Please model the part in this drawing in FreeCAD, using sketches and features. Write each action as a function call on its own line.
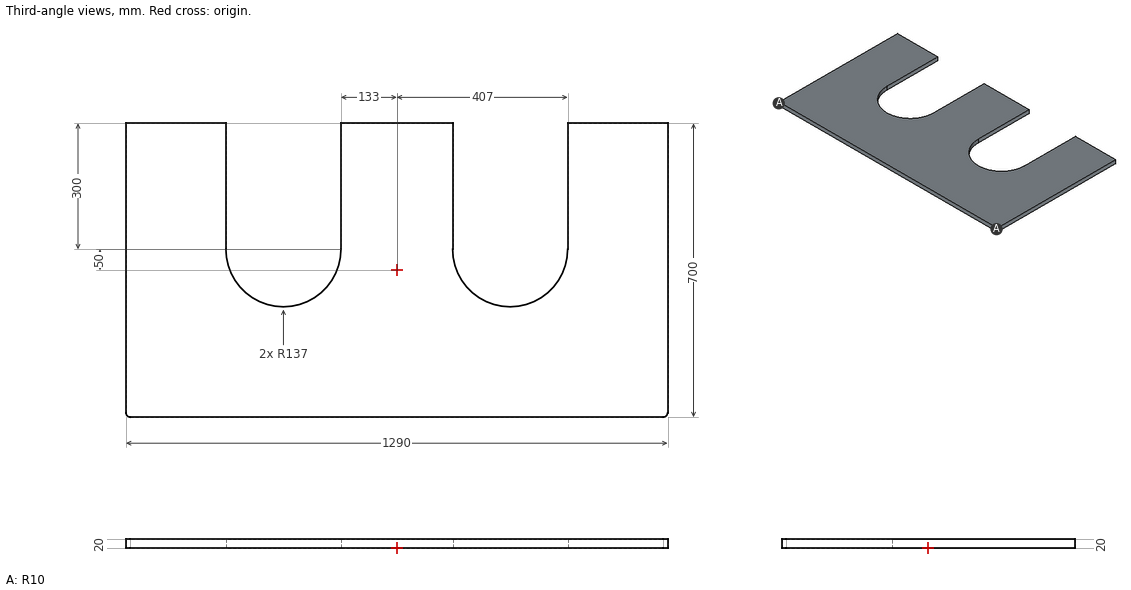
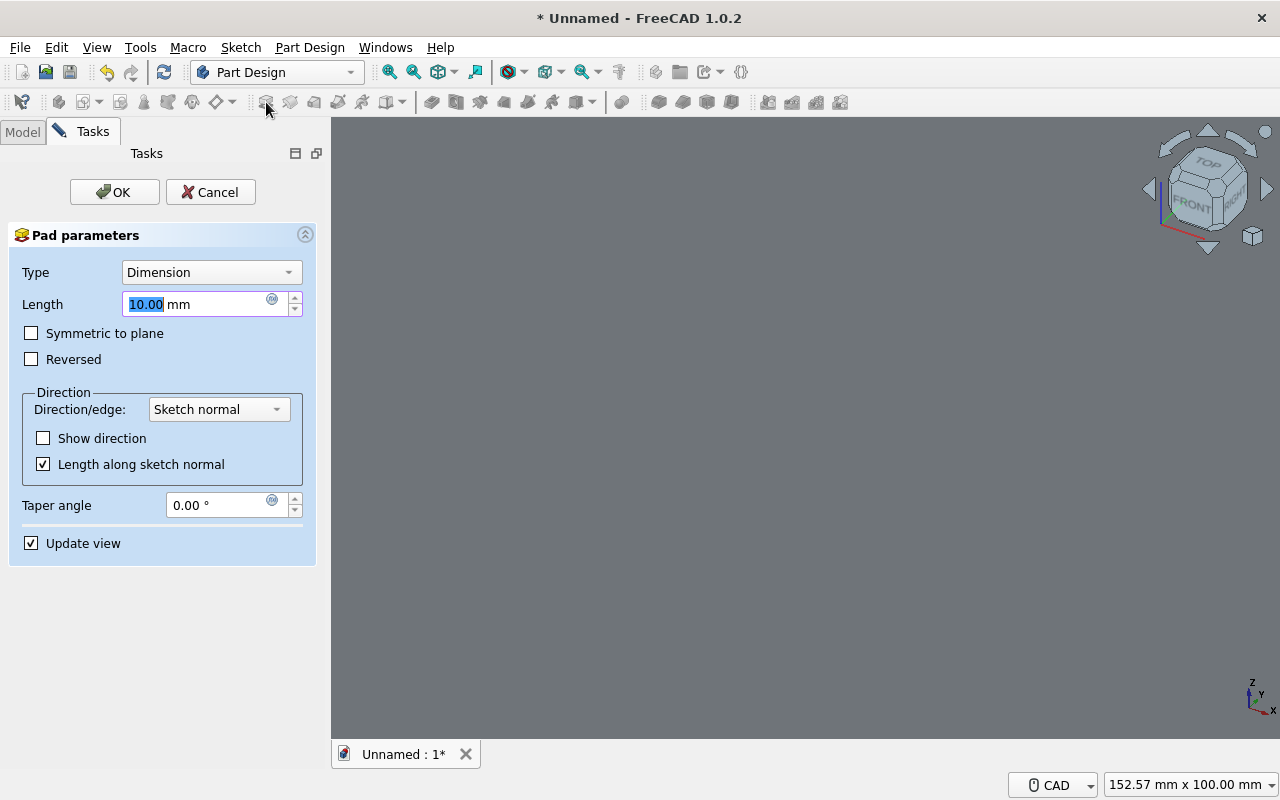
text(20)
key(Tab)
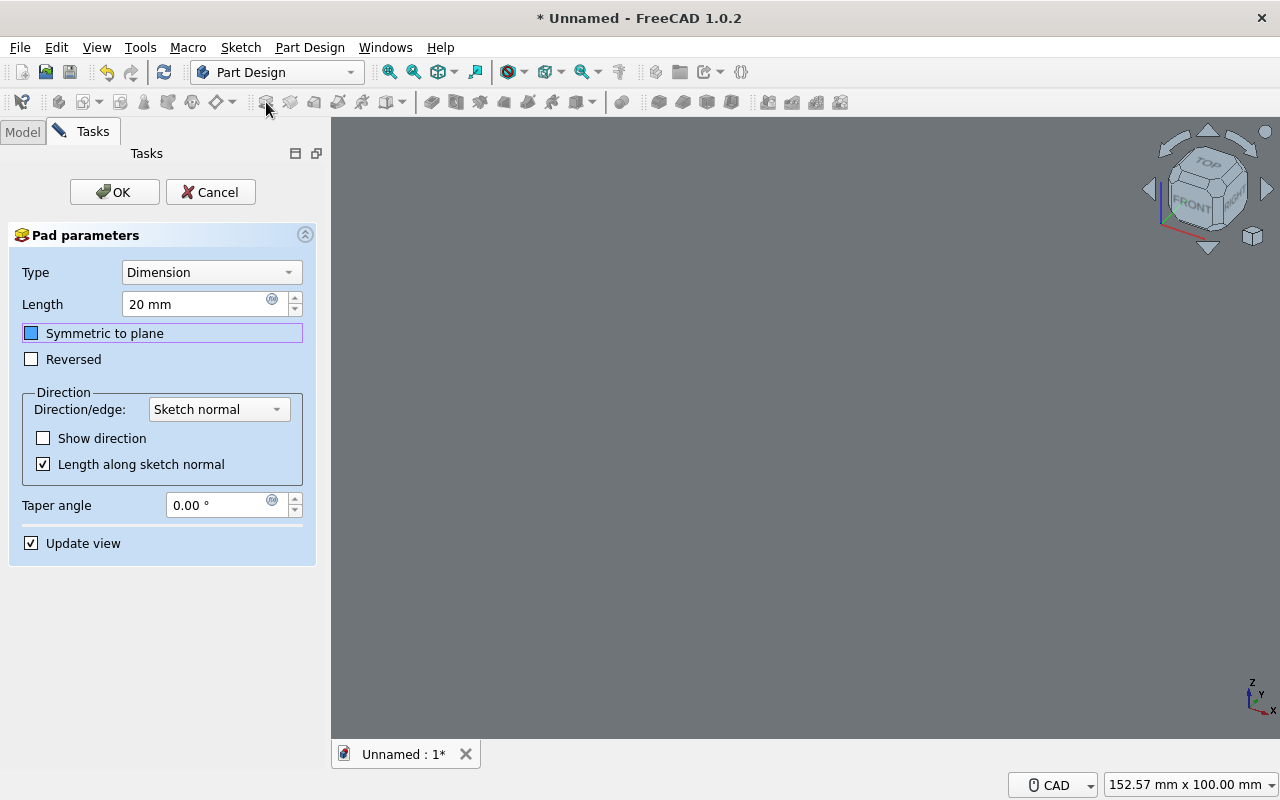
click(115, 192)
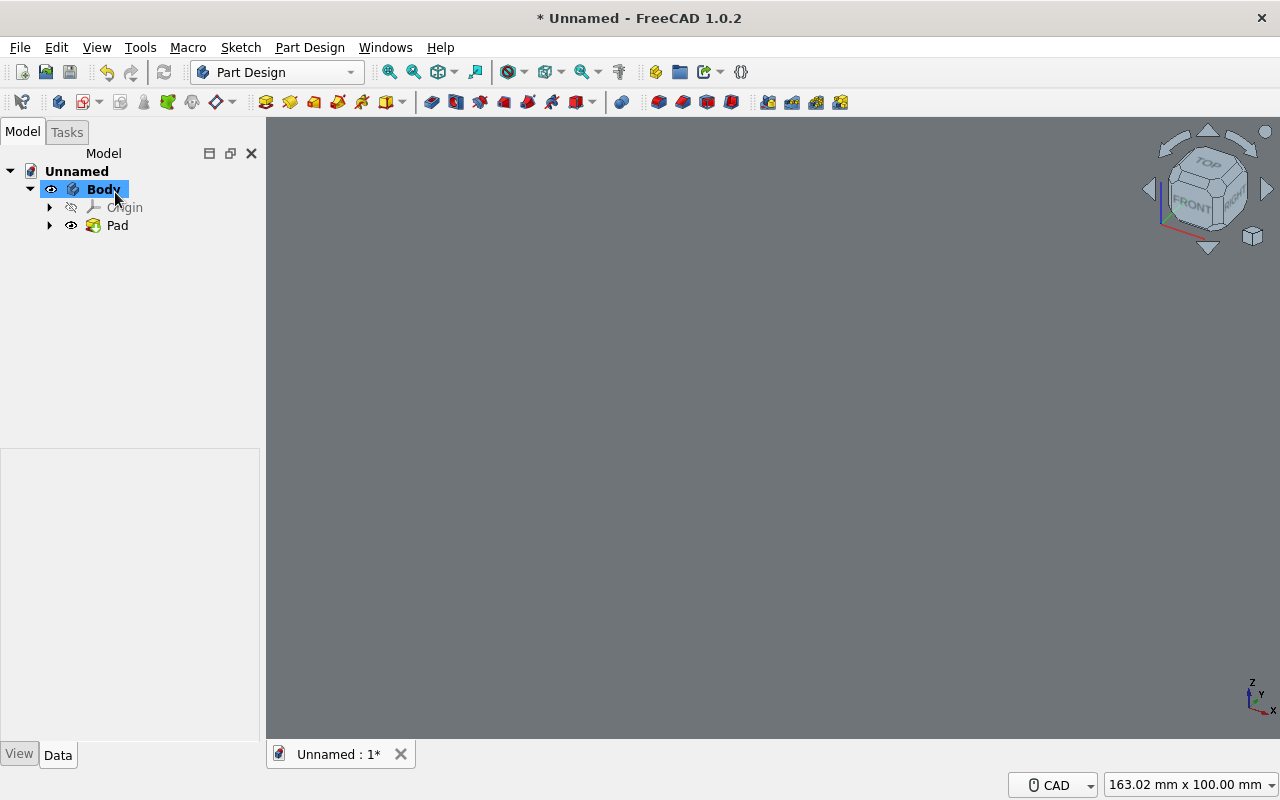
key(v)
key(f)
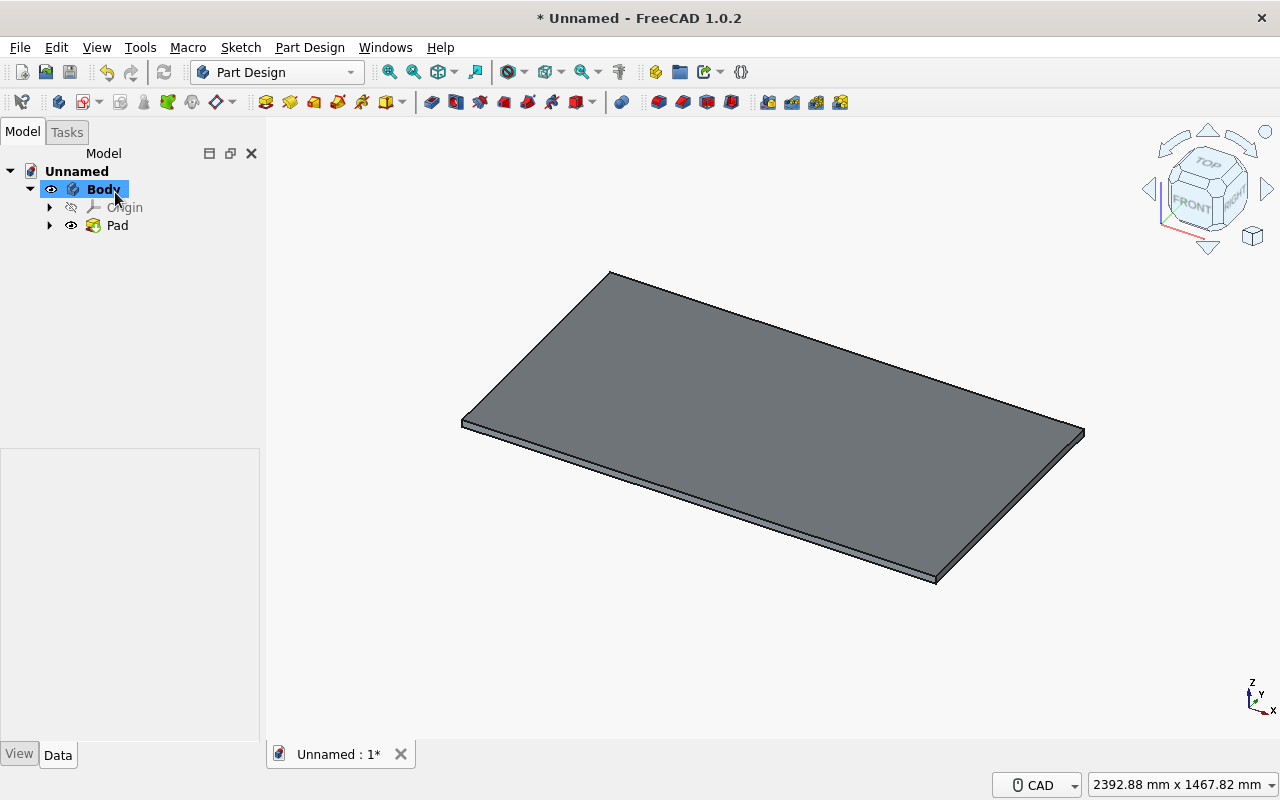
click(841, 446)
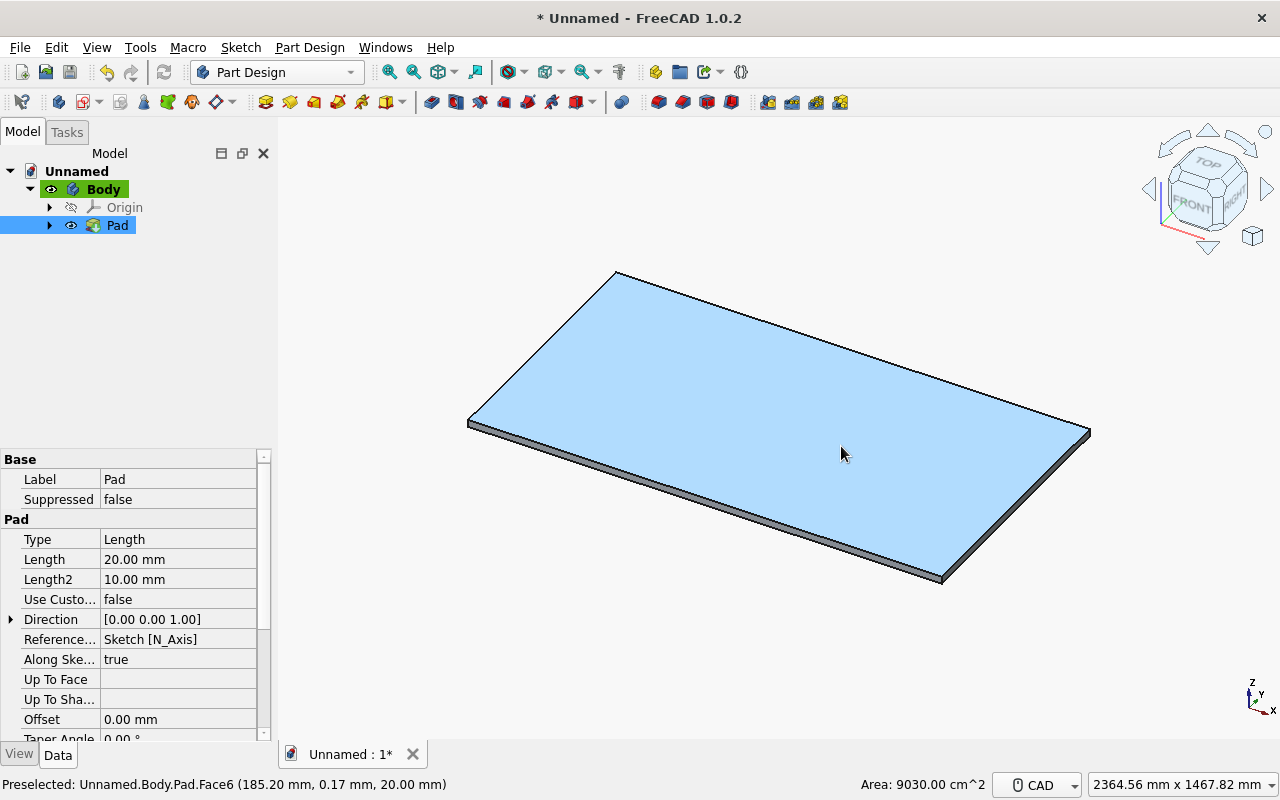
click(84, 102)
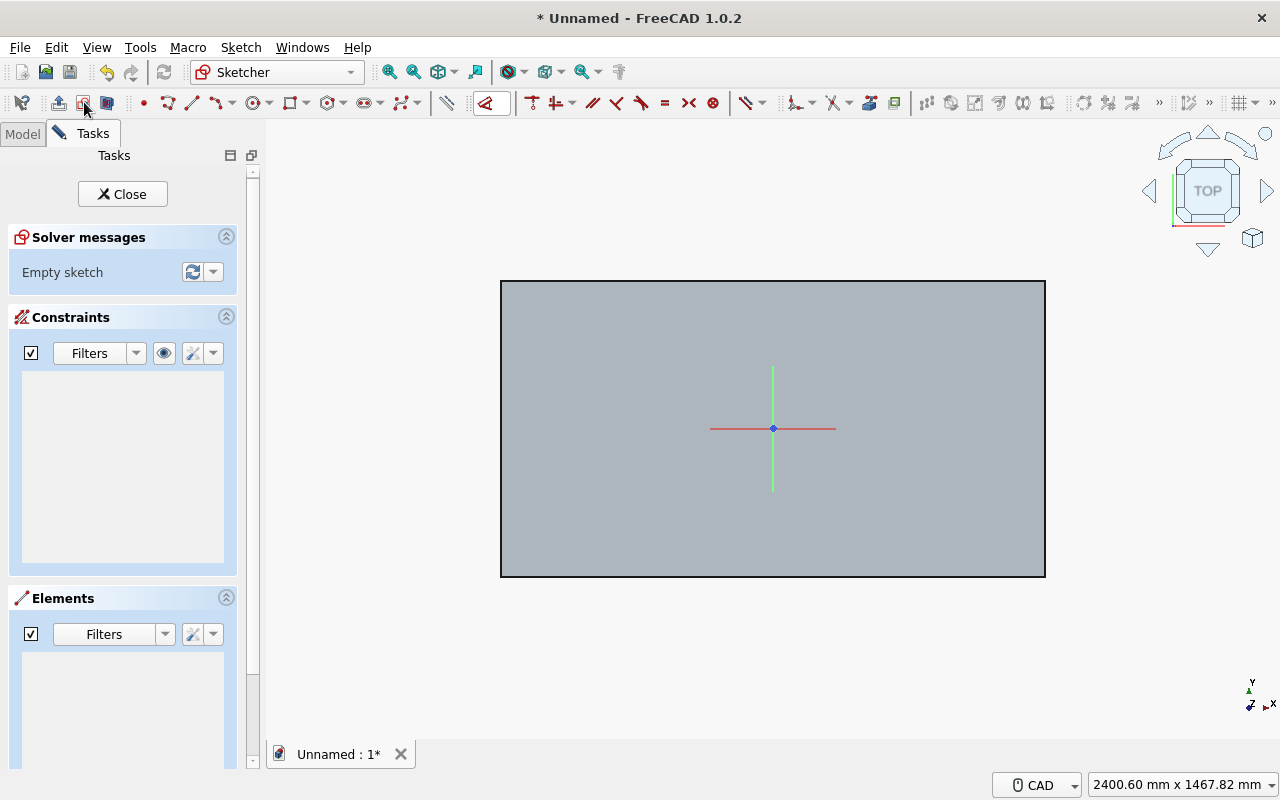
scroll(856, 306, up, 3)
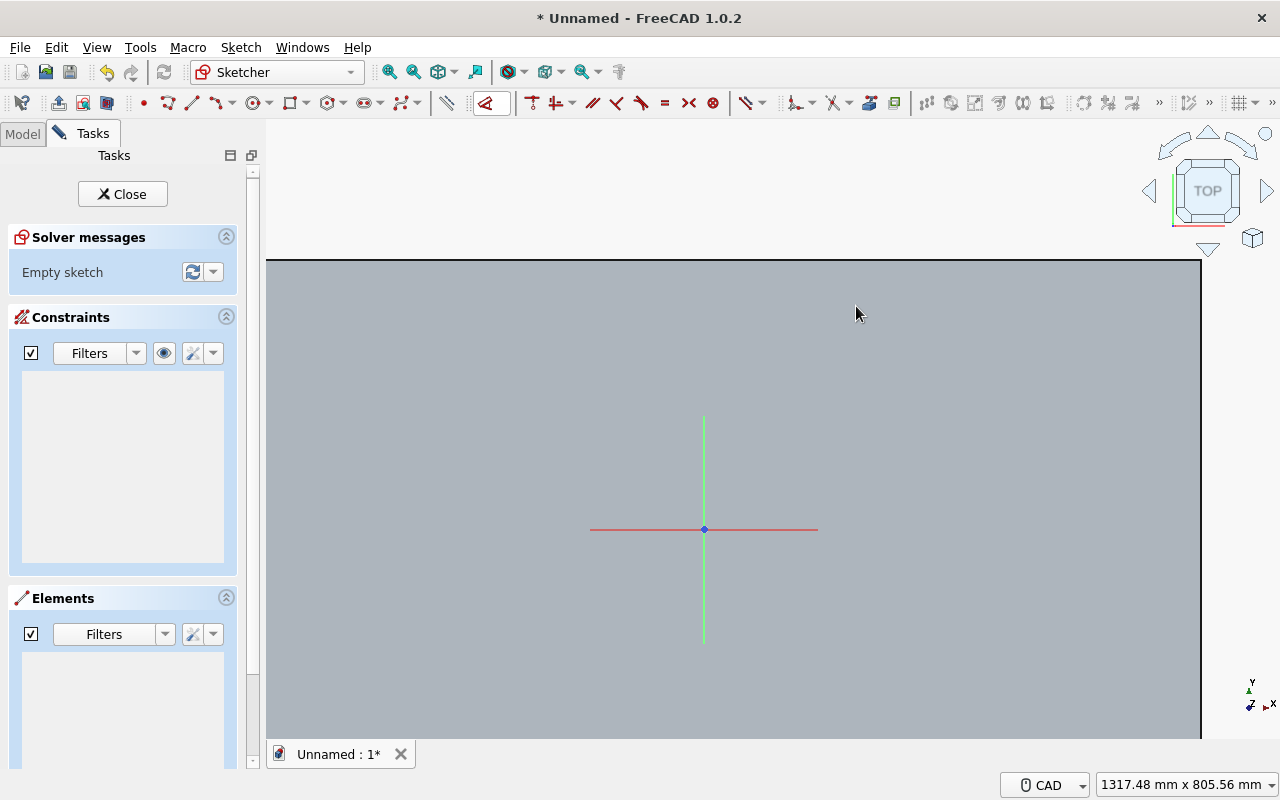
key(g)
key(m)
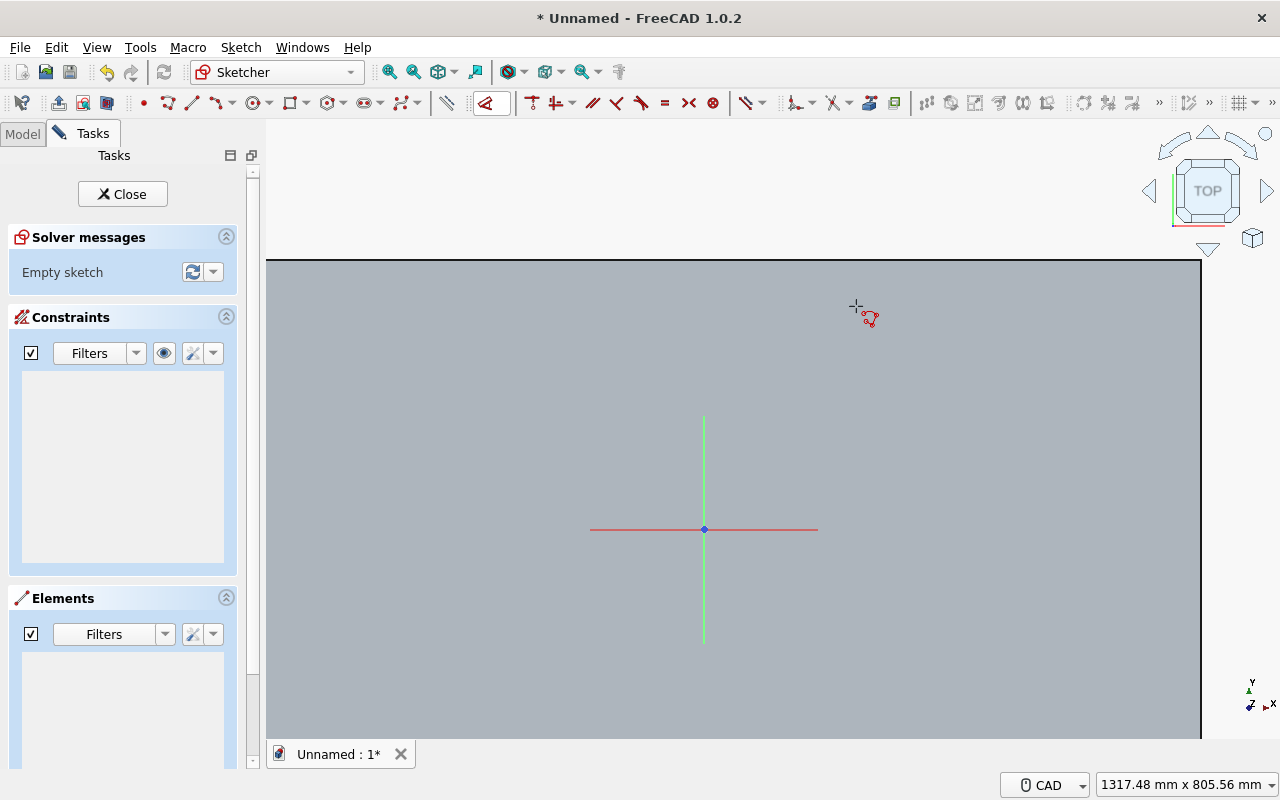
click(602, 491)
click(602, 260)
click(391, 260)
click(391, 491)
right_click(391, 491)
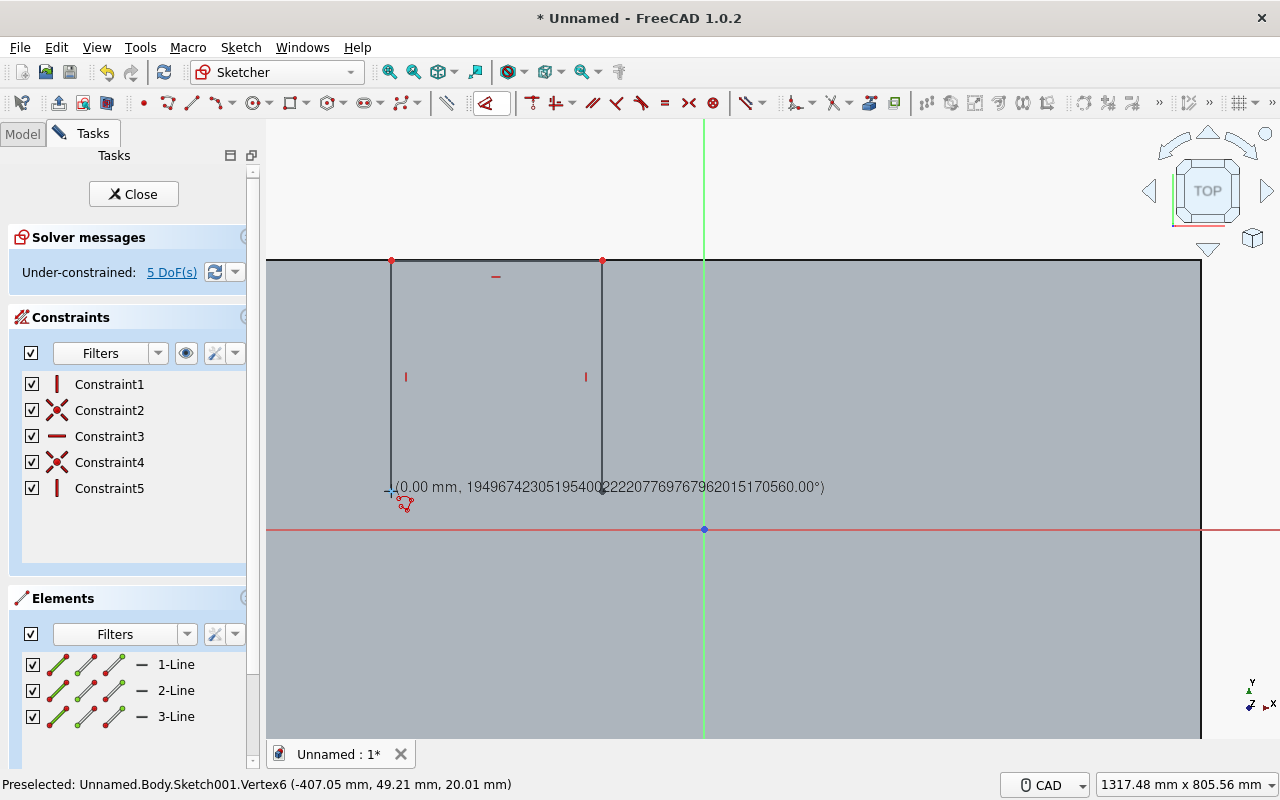
key(g)
key(3)
key(a)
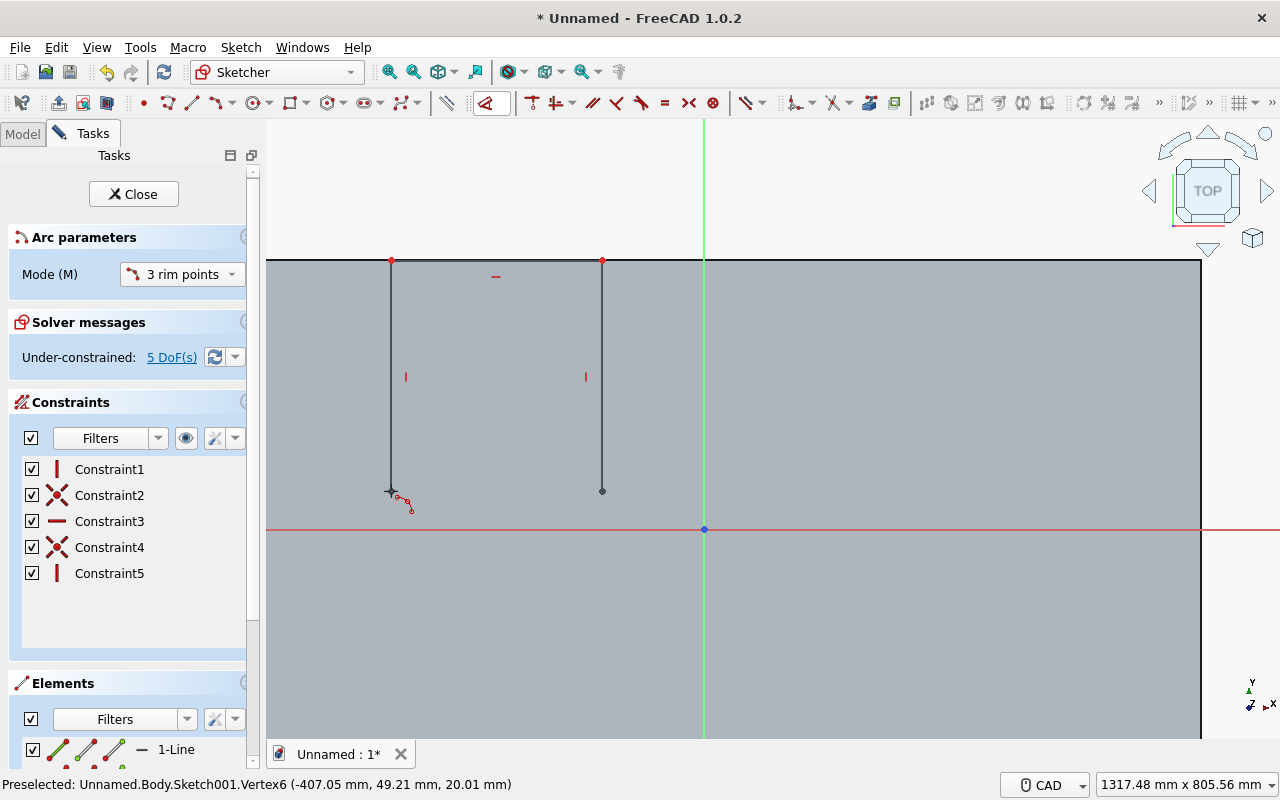
click(391, 492)
click(602, 492)
click(496, 597)